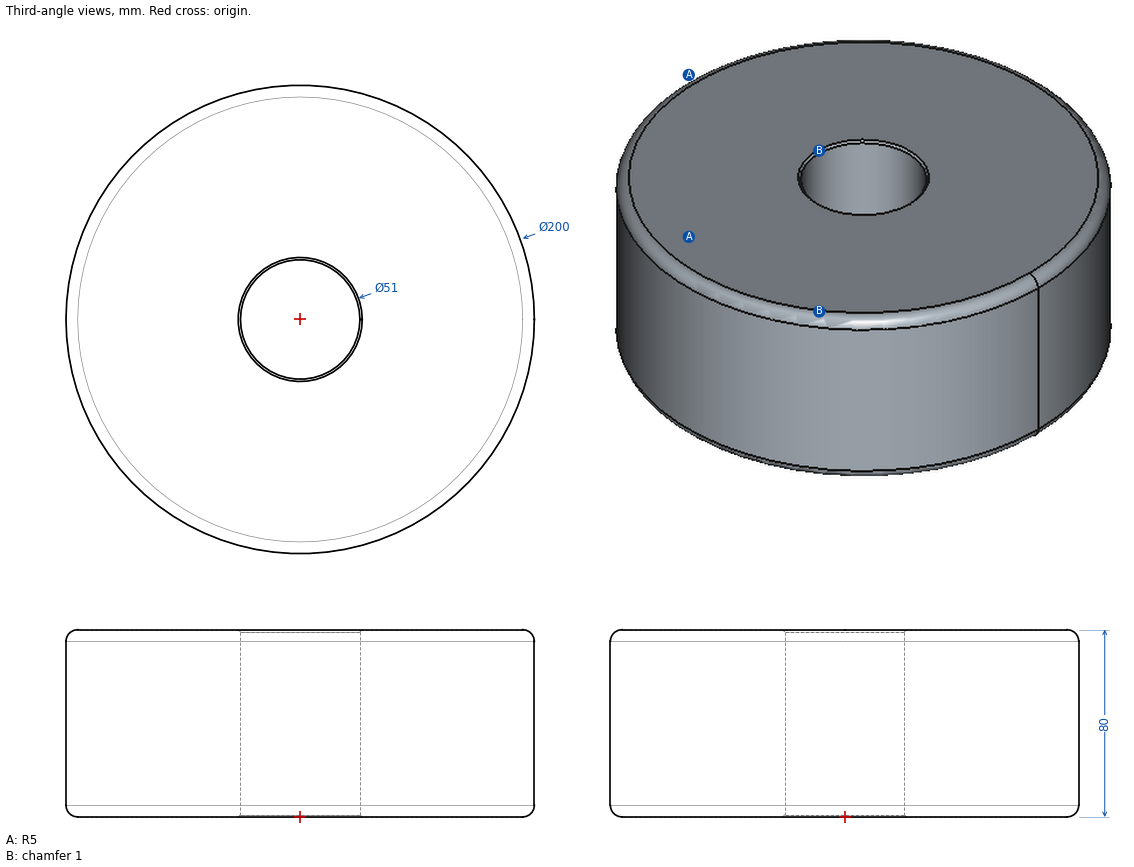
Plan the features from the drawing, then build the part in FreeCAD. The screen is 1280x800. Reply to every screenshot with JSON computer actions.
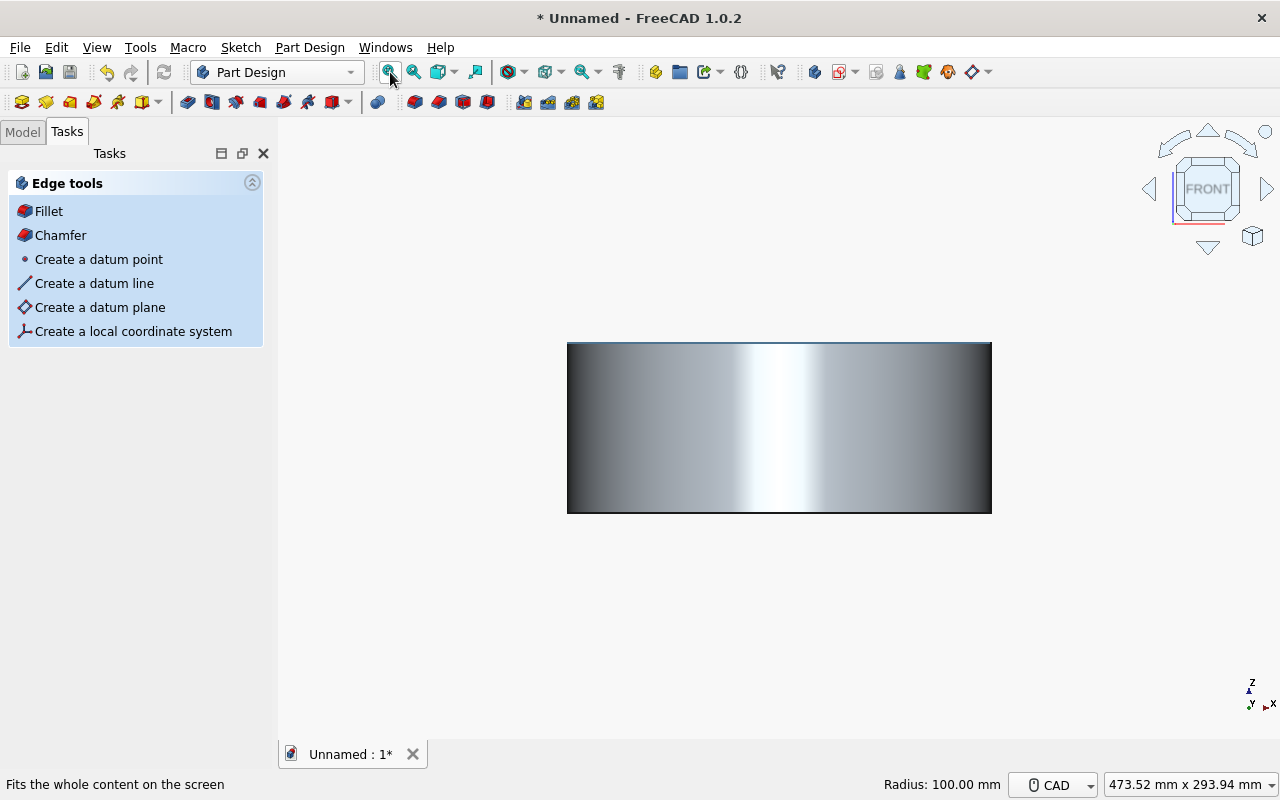
{"action": "left_click", "coordinate": [608, 512], "text": "ctrl"}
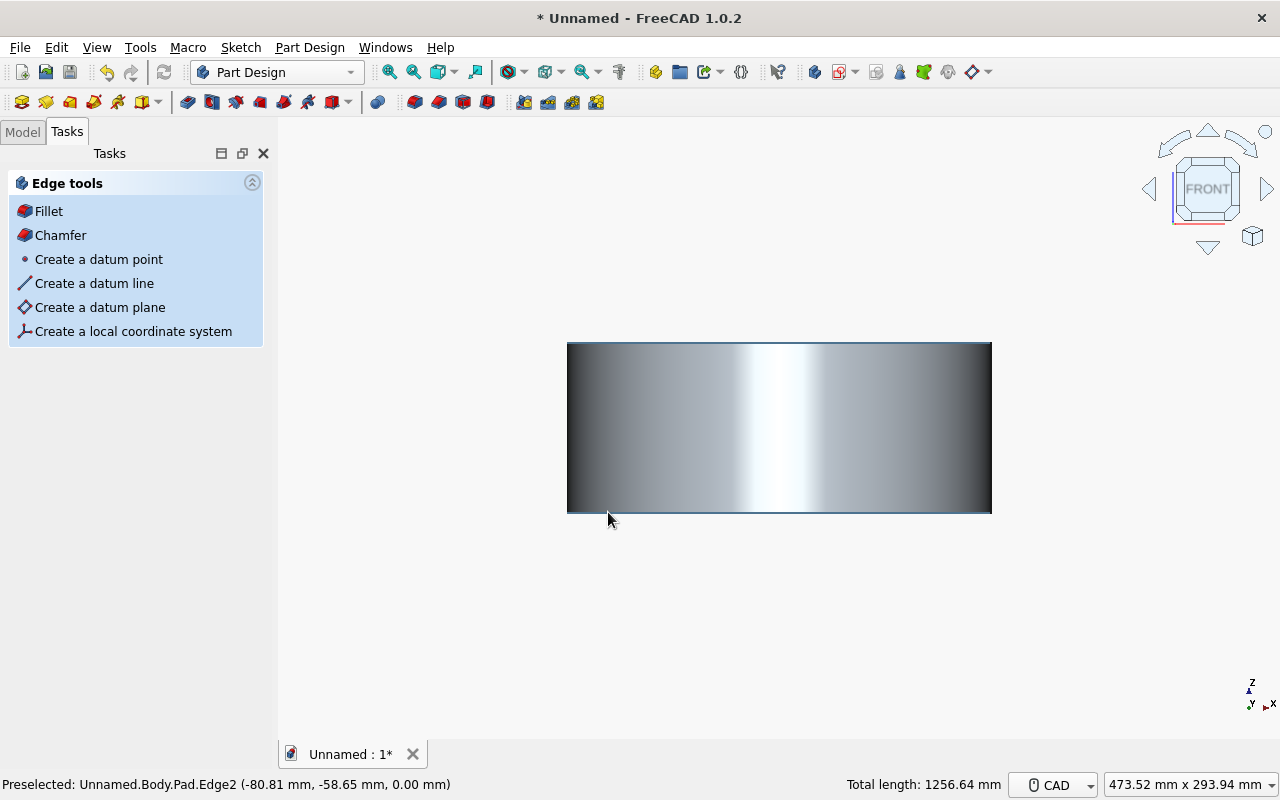
{"action": "left_click", "coordinate": [416, 102]}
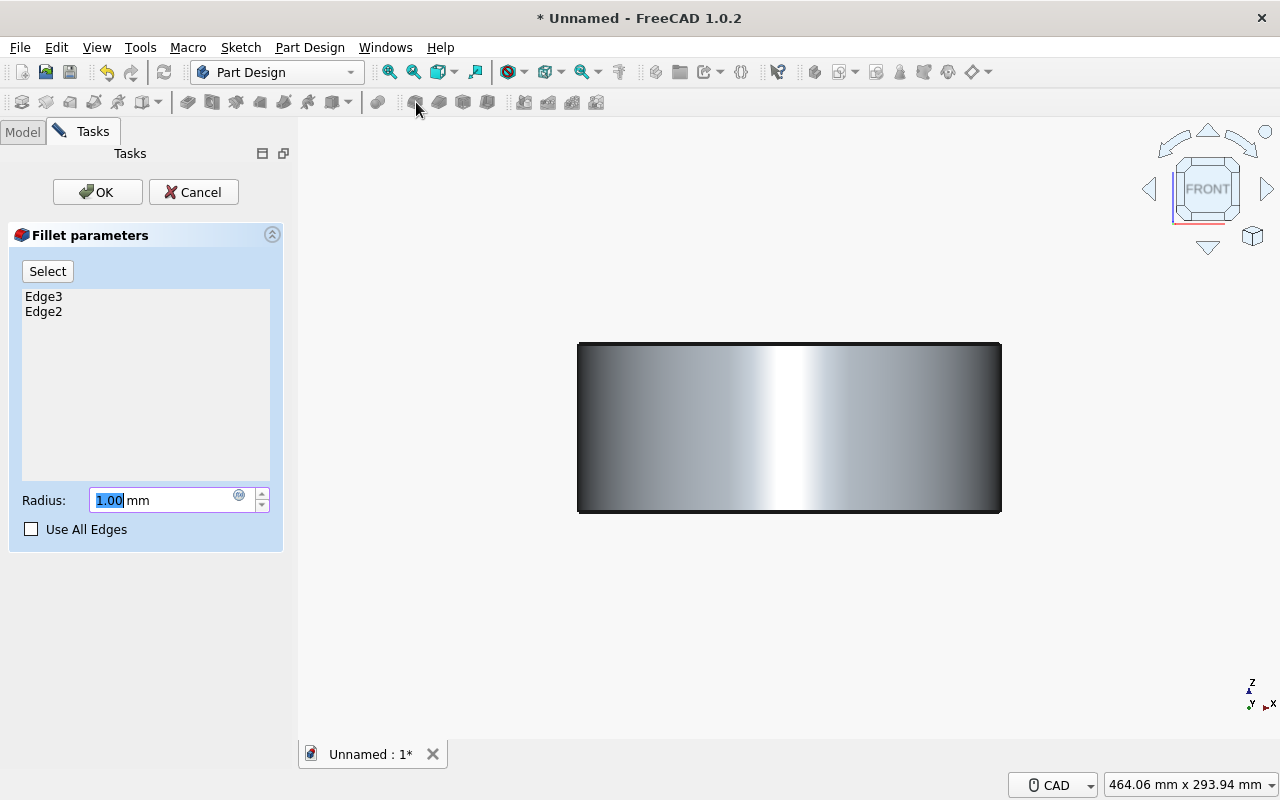
{"action": "type", "text": "5"}
{"action": "key", "text": "Tab"}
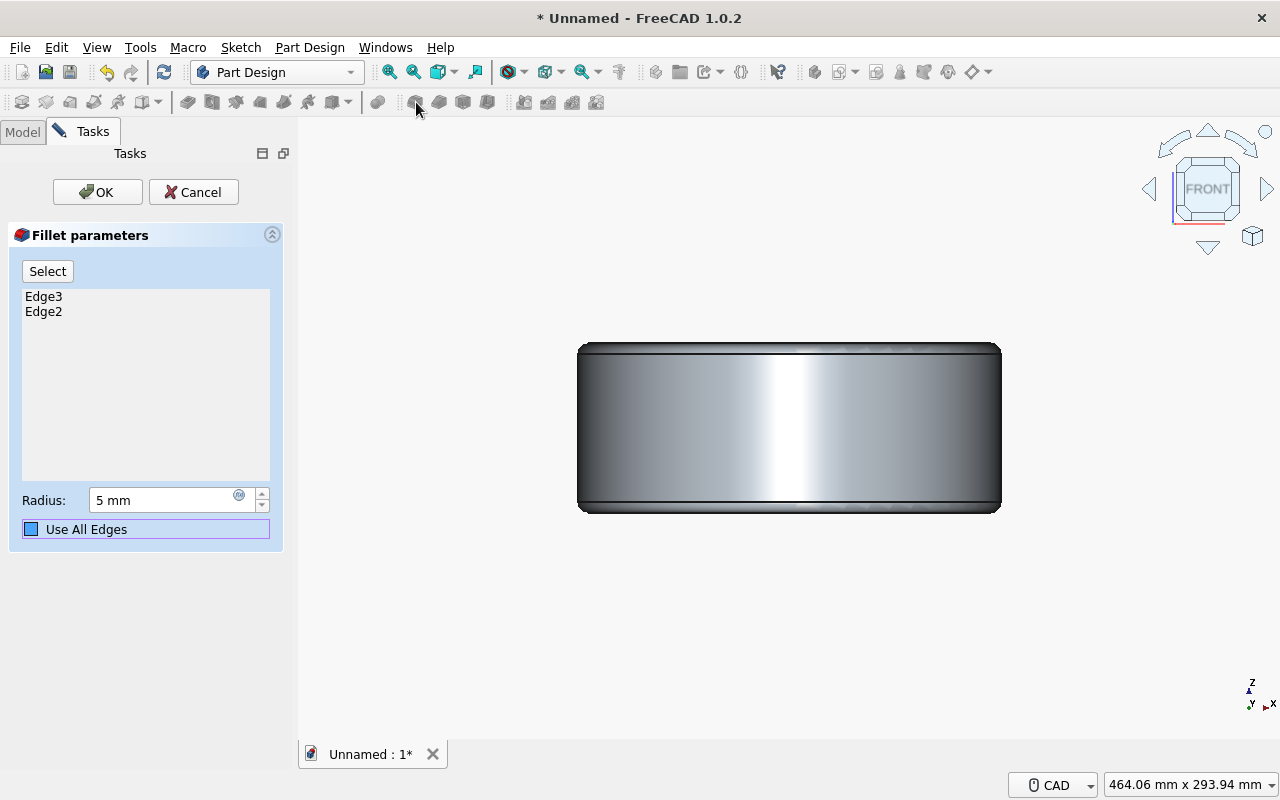
{"action": "left_click", "coordinate": [98, 192]}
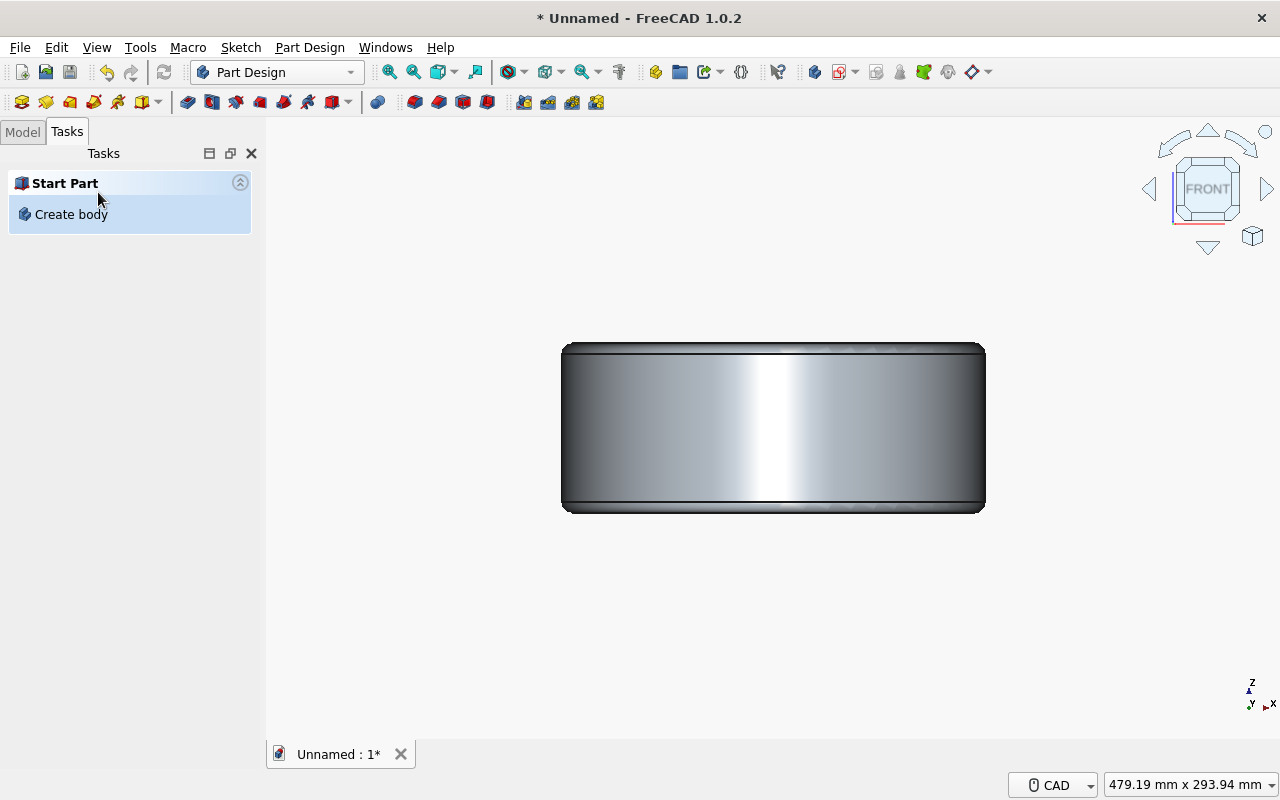
{"action": "left_click", "coordinate": [390, 72]}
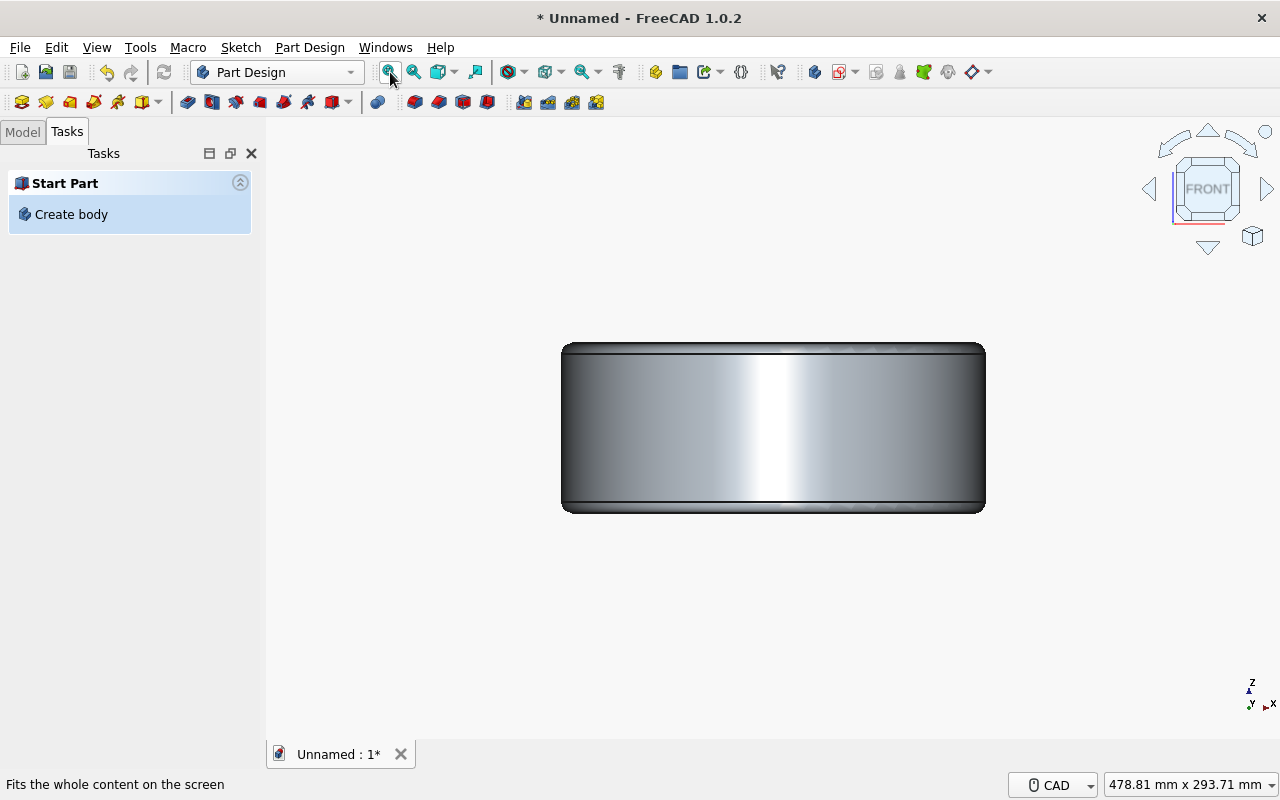
{"action": "key", "text": "0"}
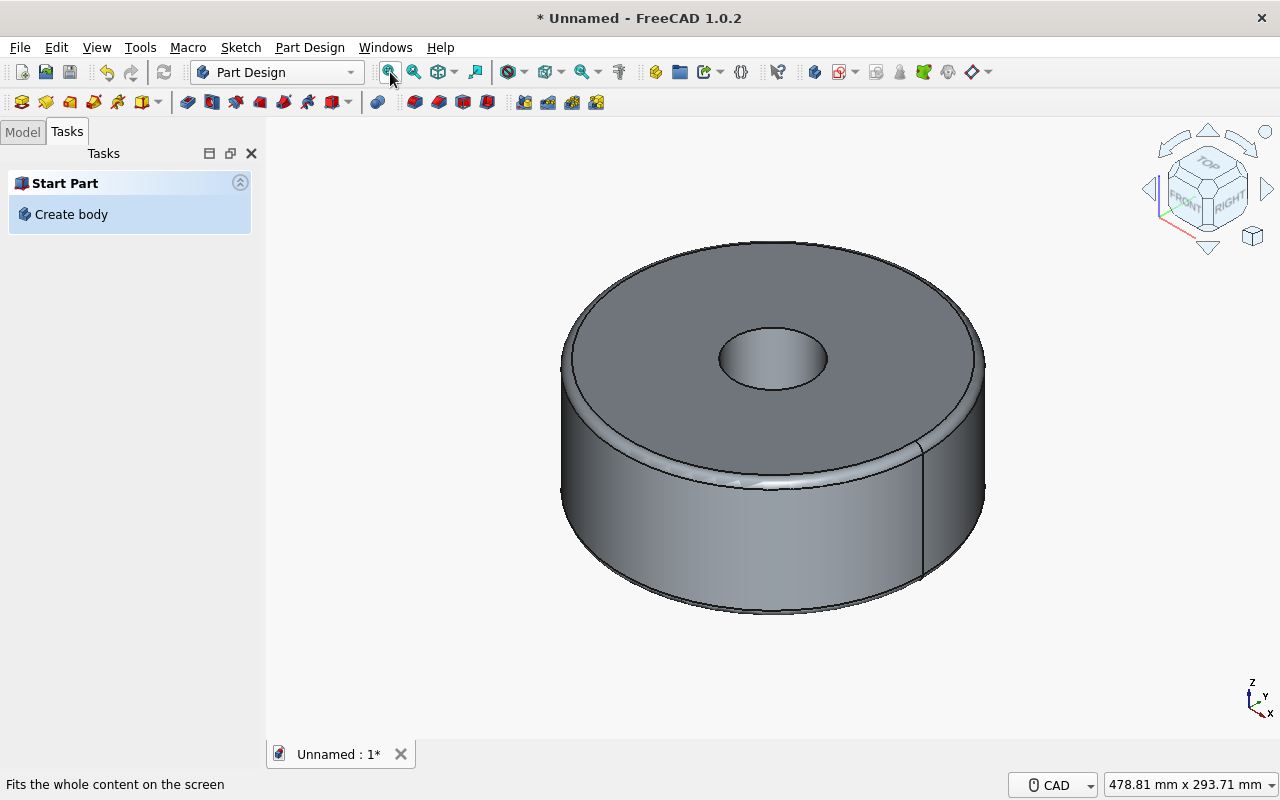
{"action": "left_click", "coordinate": [735, 336]}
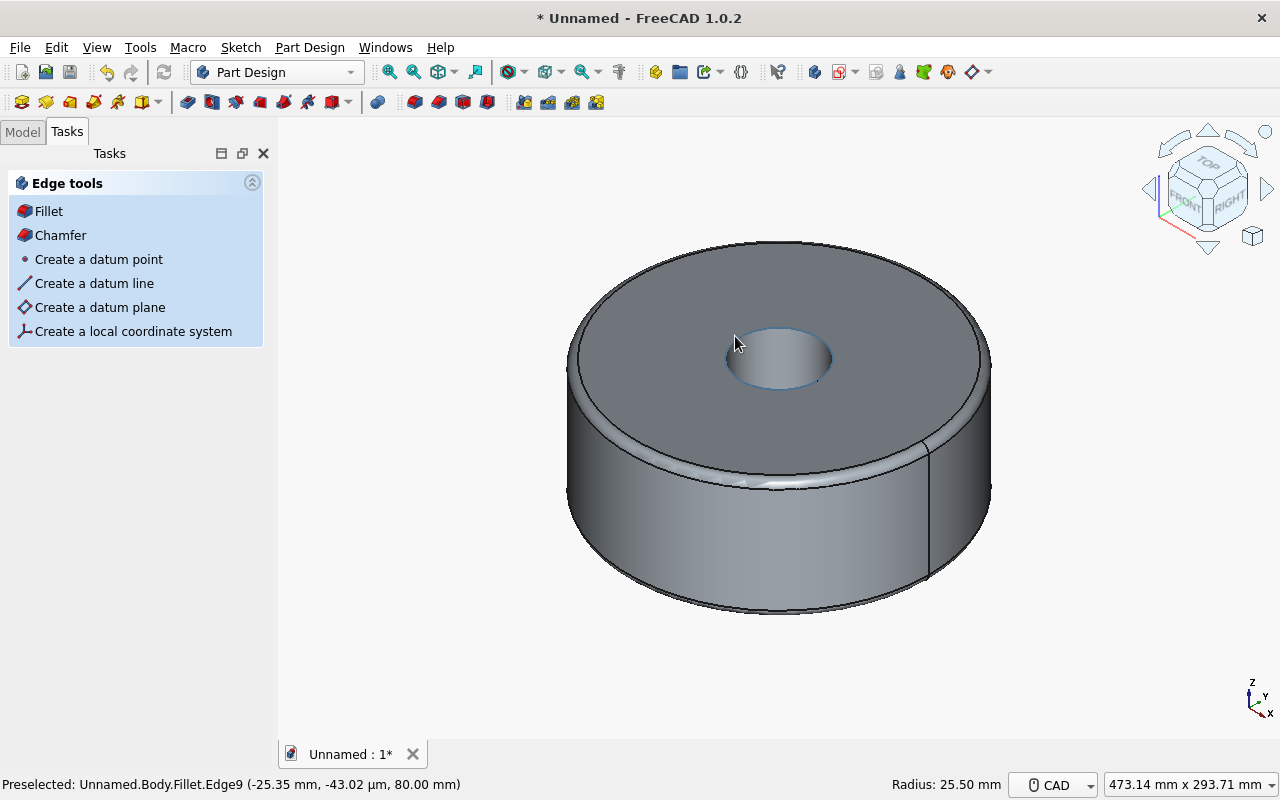
{"action": "key", "text": "2"}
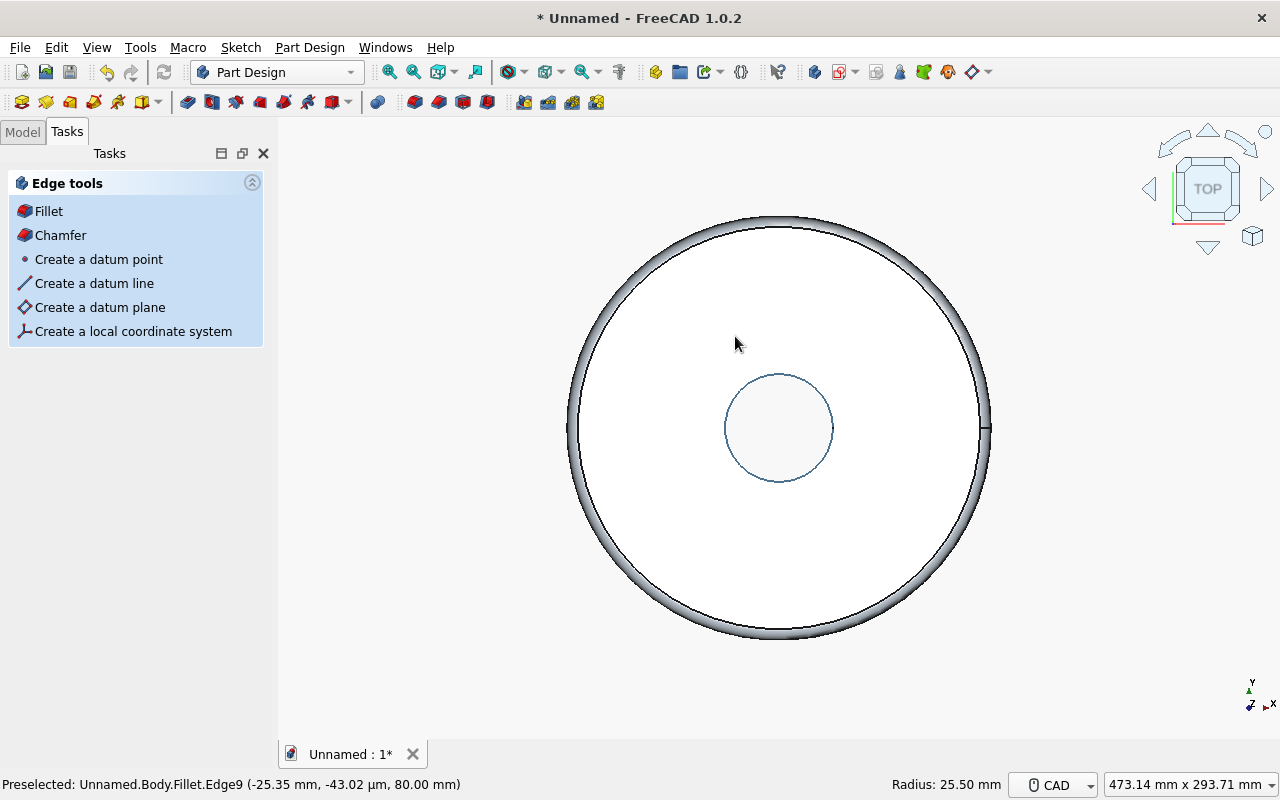
{"action": "key", "text": "1"}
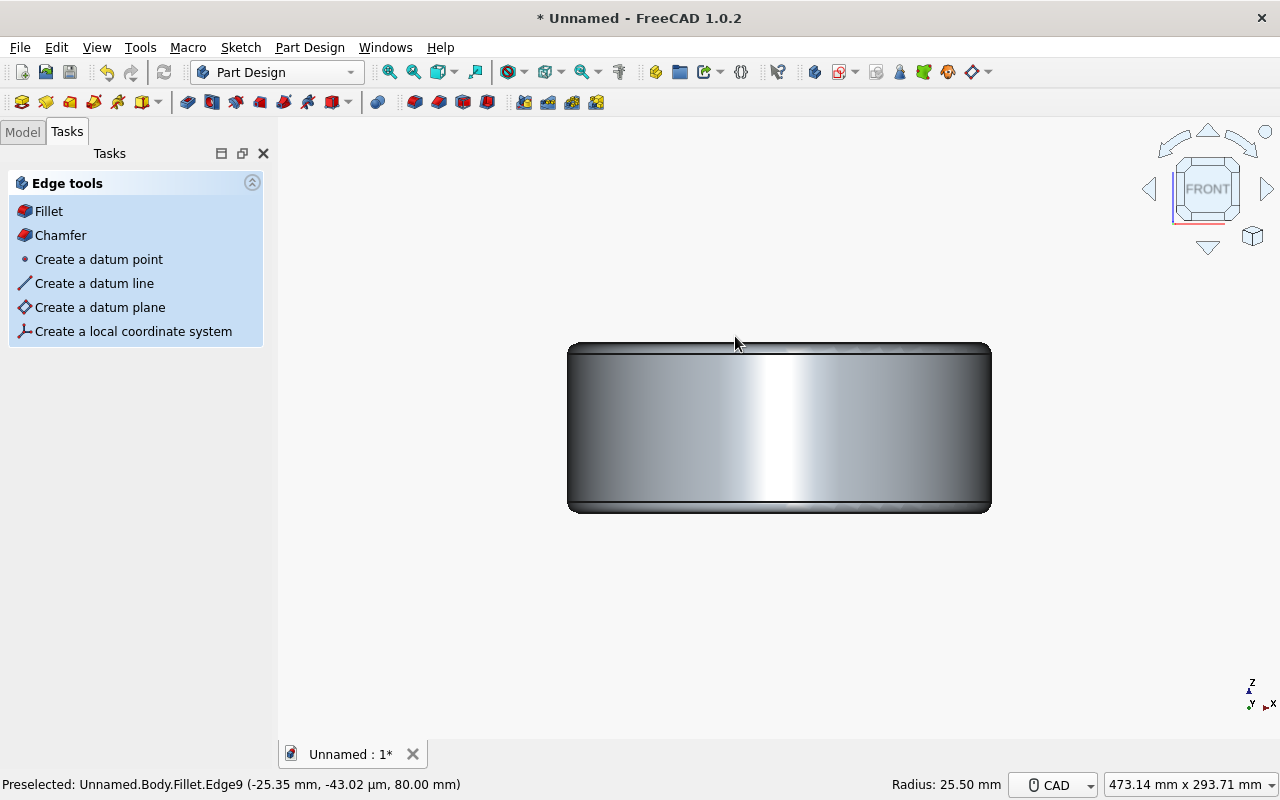
{"action": "left_click", "coordinate": [390, 72]}